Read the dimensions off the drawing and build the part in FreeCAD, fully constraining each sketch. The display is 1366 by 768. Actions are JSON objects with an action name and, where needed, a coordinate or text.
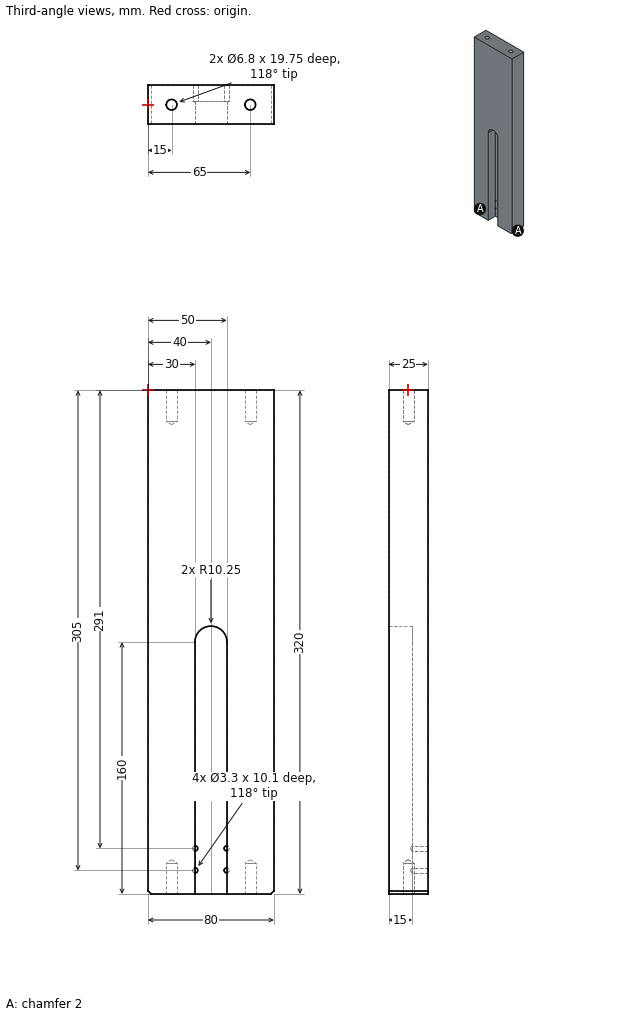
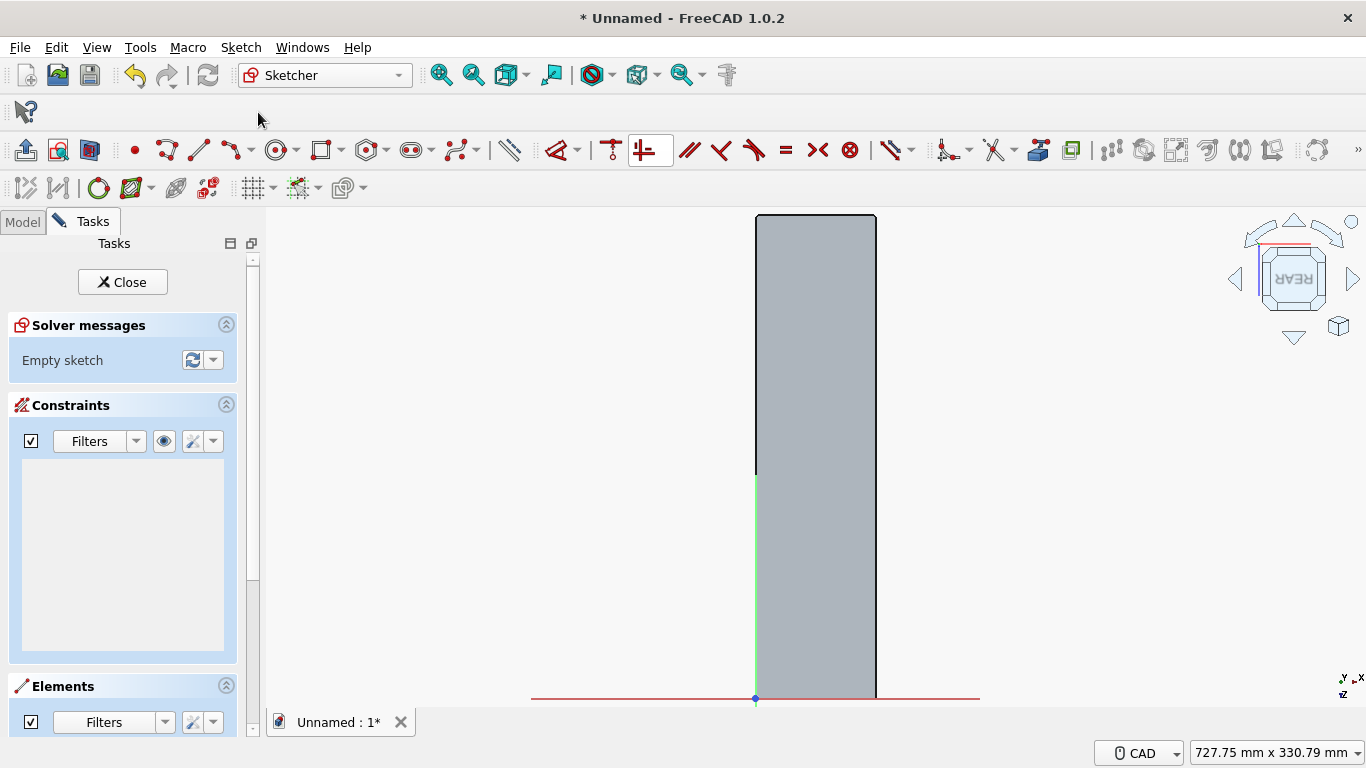
{"action": "scroll", "coordinate": [748, 457], "scroll_direction": "down", "scroll_amount": 5}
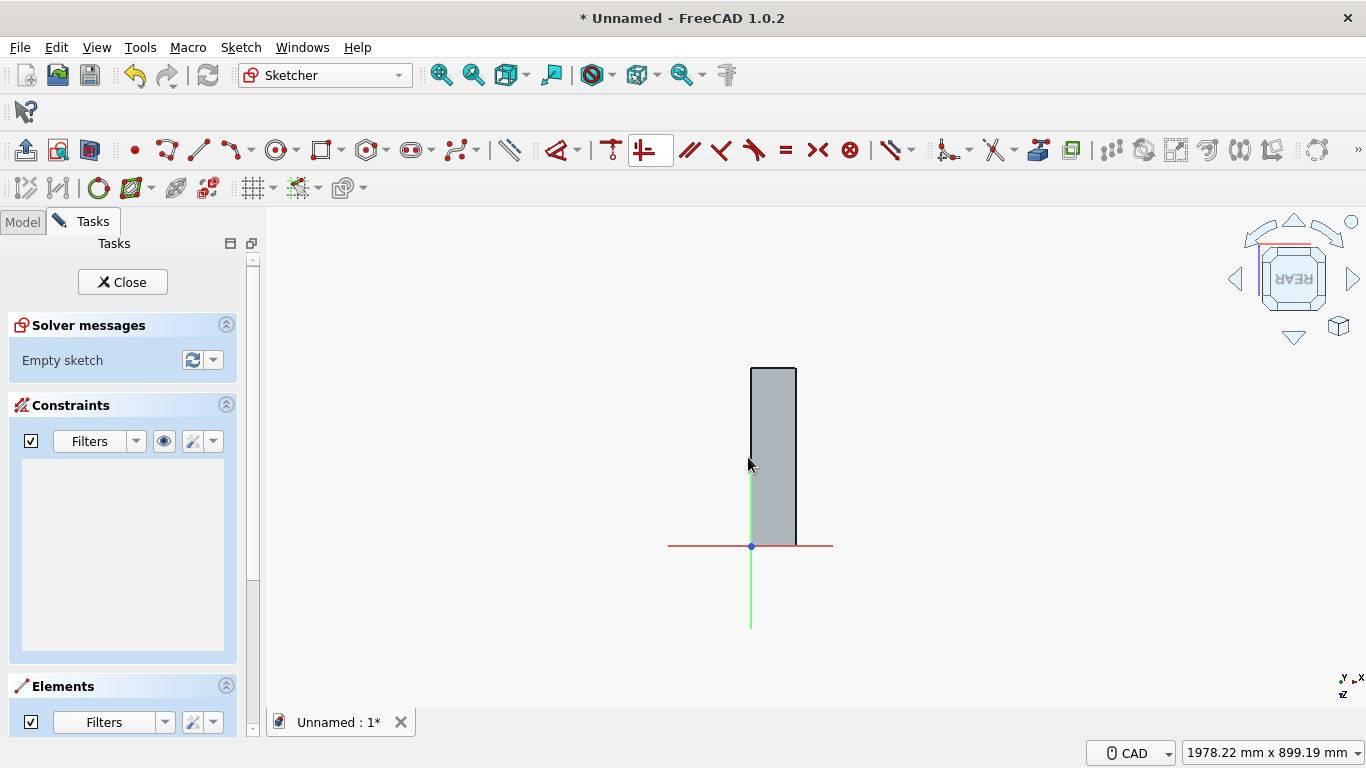
{"action": "scroll", "coordinate": [775, 377], "scroll_direction": "up", "scroll_amount": 15}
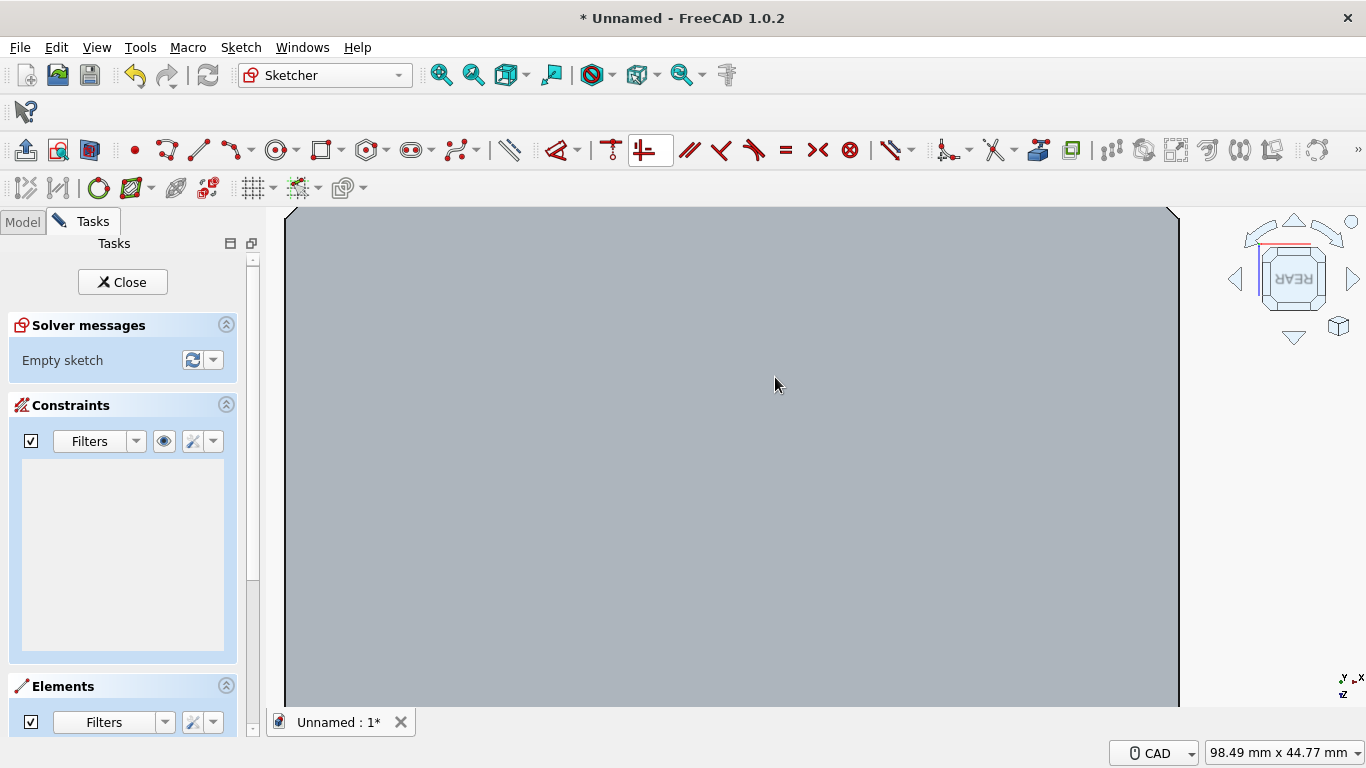
{"action": "scroll", "coordinate": [700, 413], "scroll_direction": "up", "scroll_amount": 2}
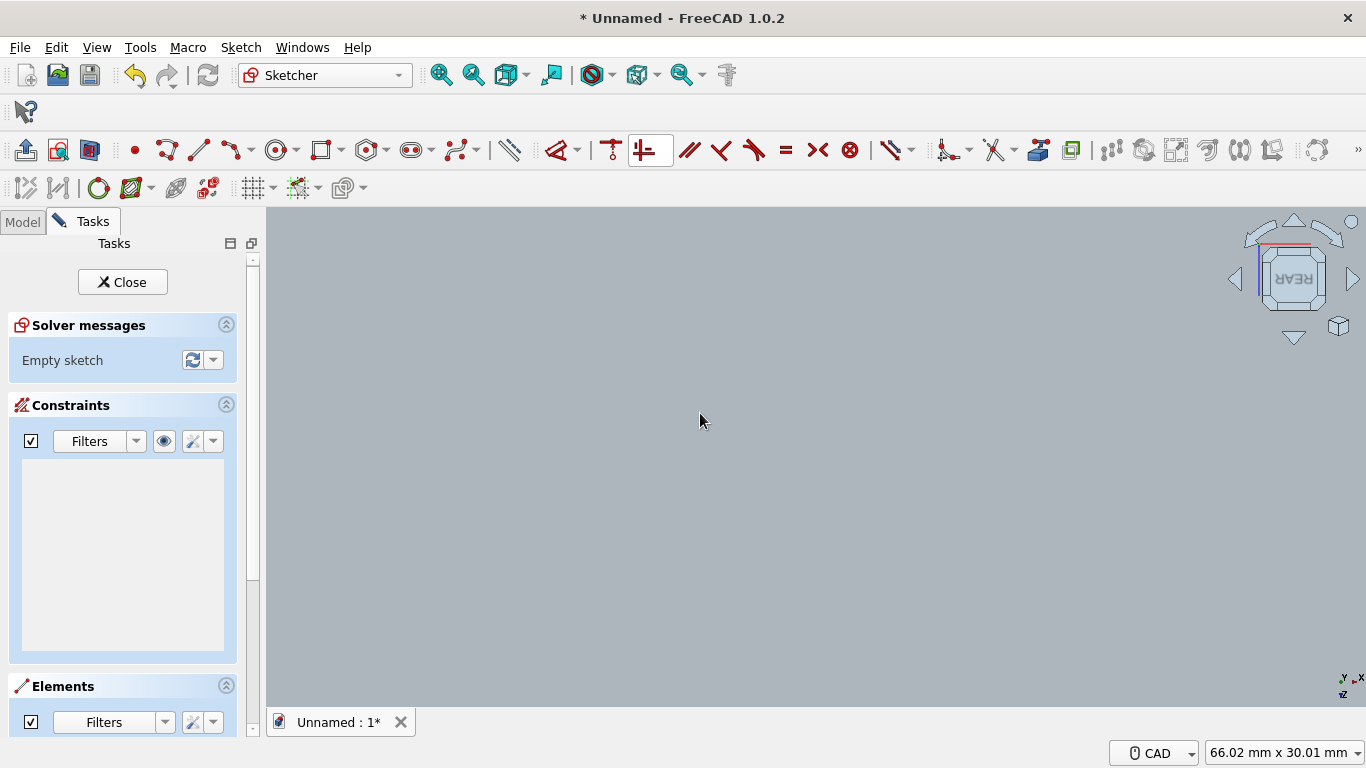
{"action": "left_click", "coordinate": [276, 150]}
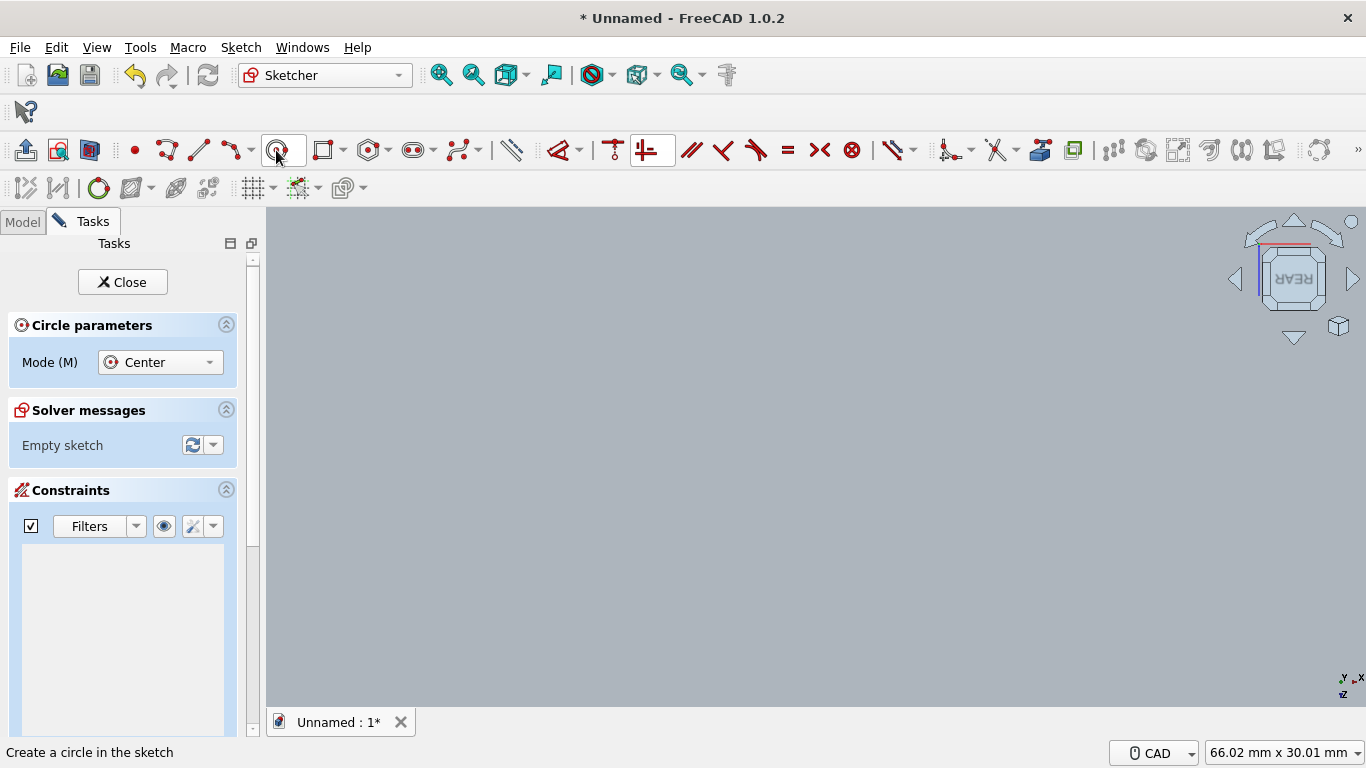
{"action": "left_click", "coordinate": [581, 340]}
{"action": "mouse_move", "coordinate": [600, 321]}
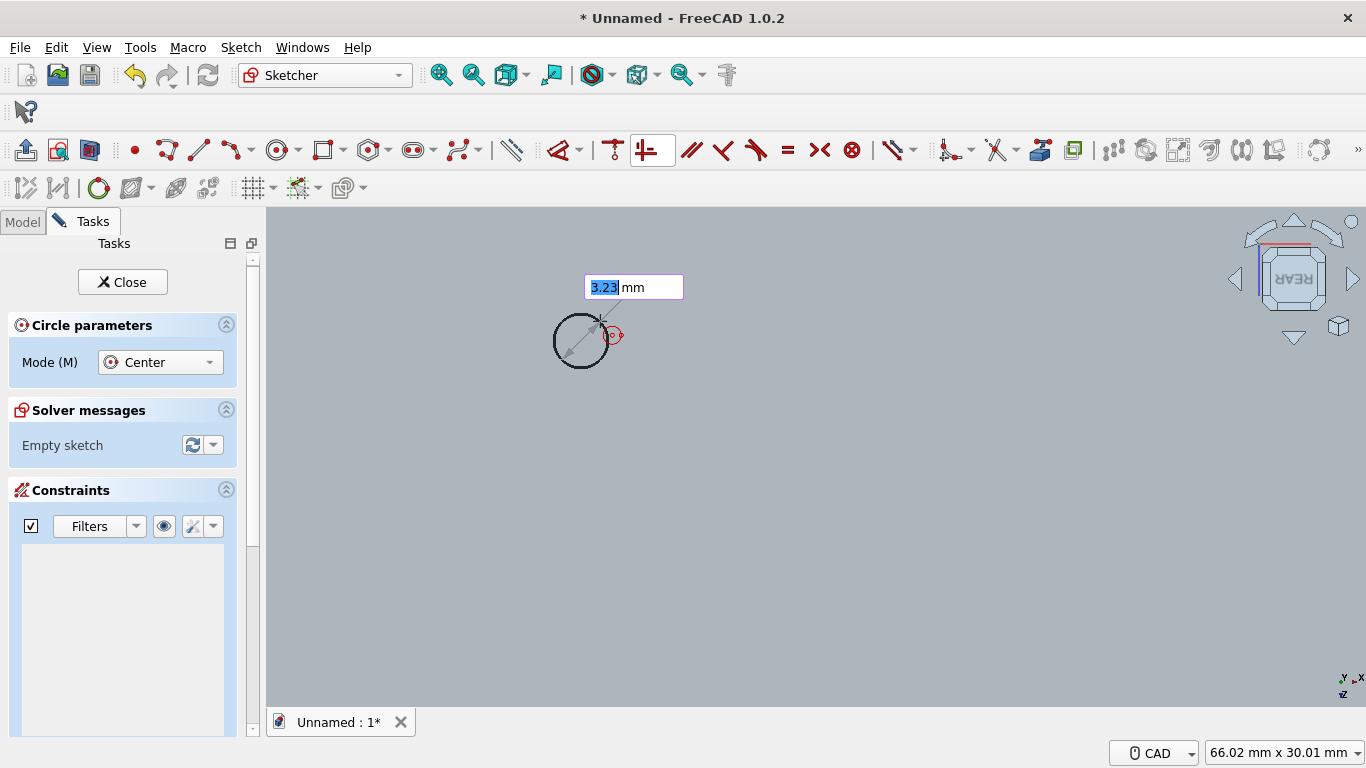
{"action": "type", "text": "3.3"}
{"action": "key", "text": "Return"}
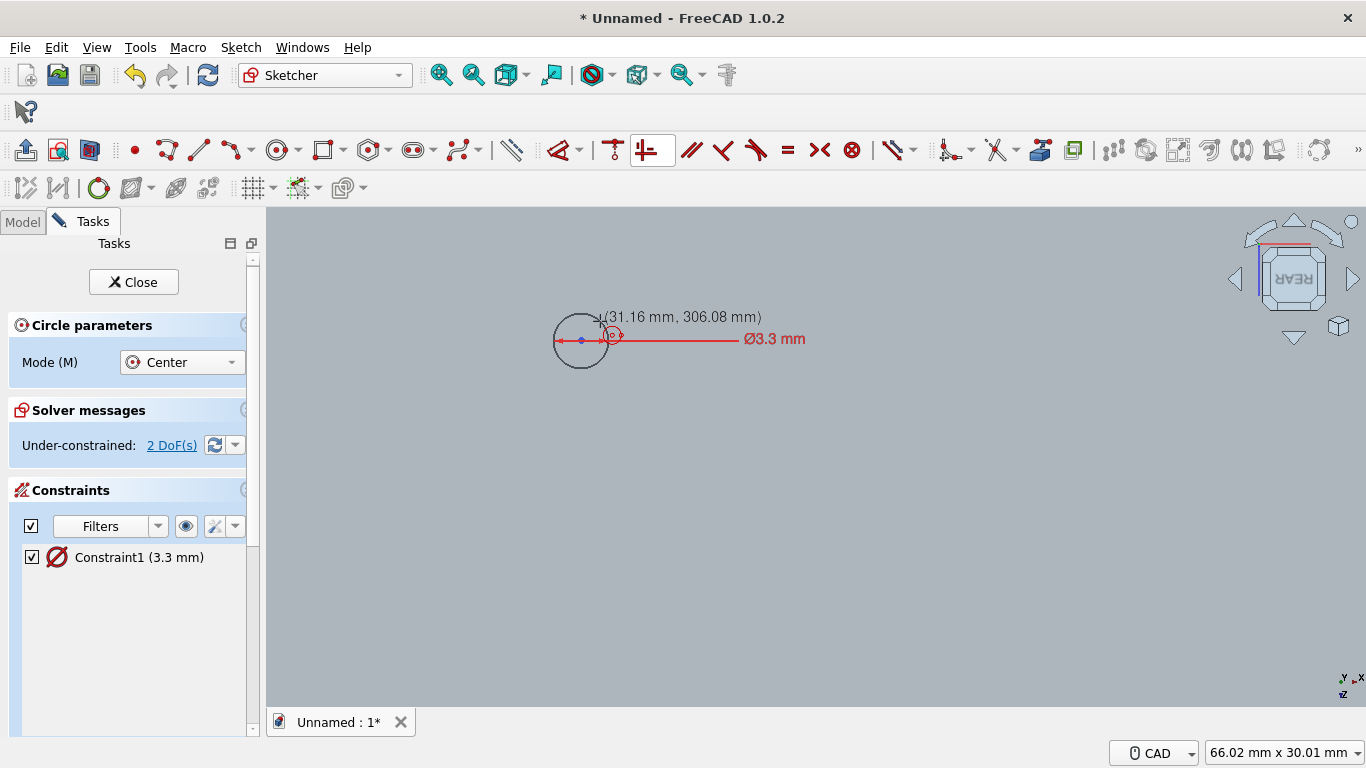
{"action": "left_click", "coordinate": [581, 573]}
{"action": "mouse_move", "coordinate": [600, 554]}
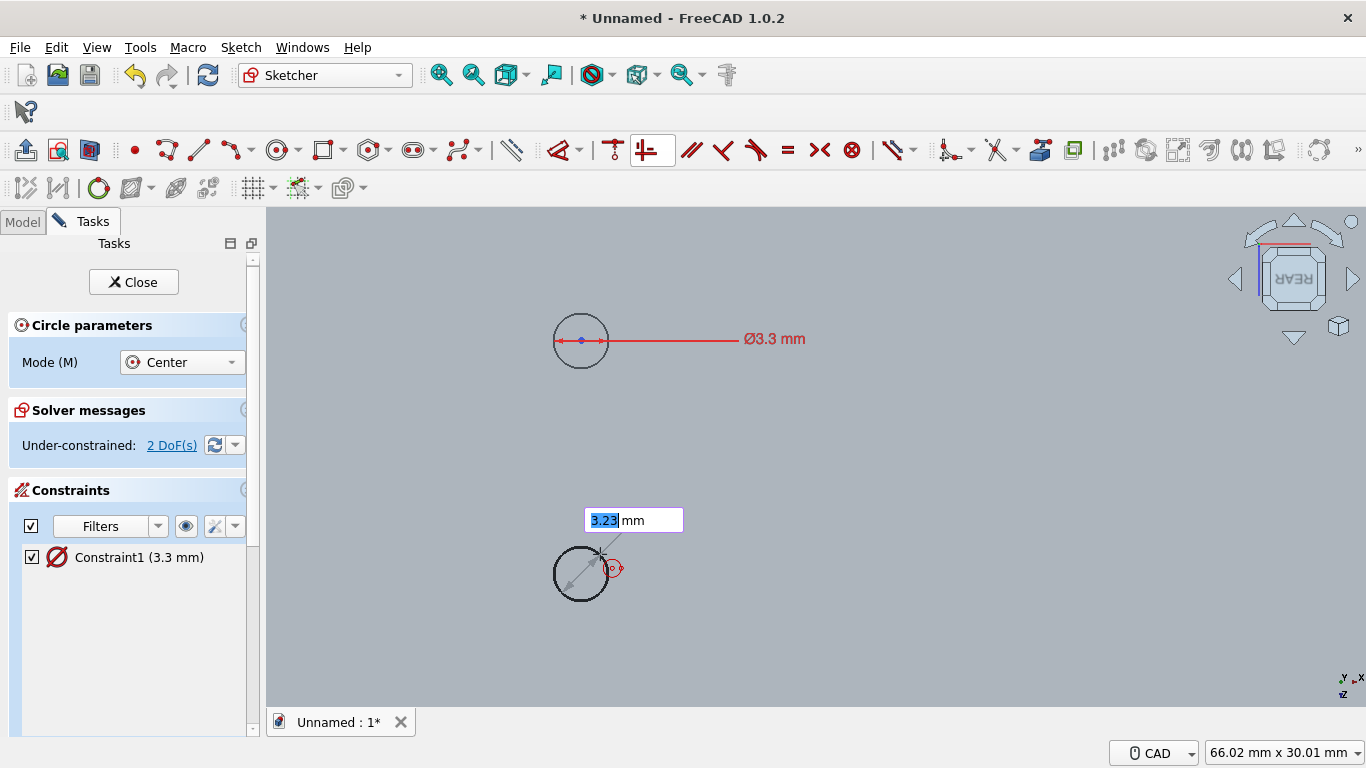
{"action": "type", "text": "3.3"}
{"action": "key", "text": "Return"}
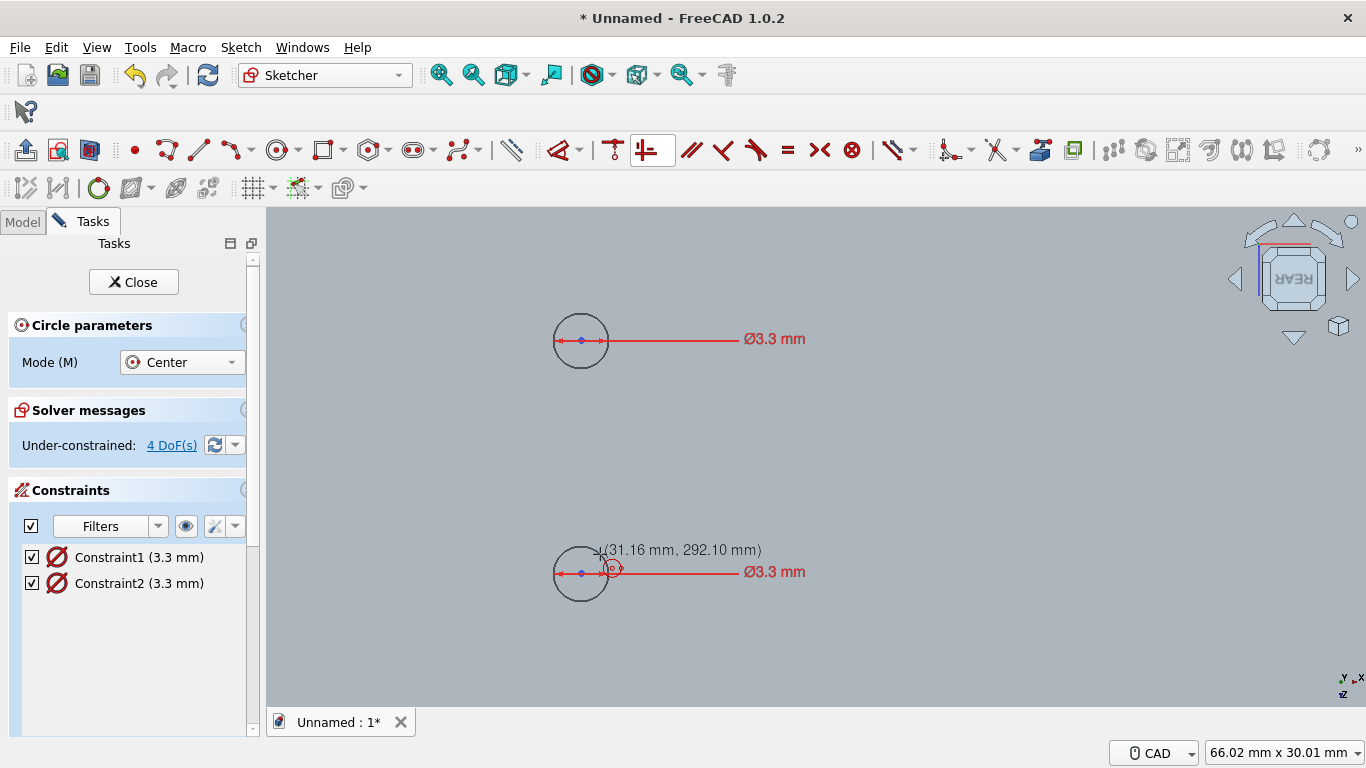
{"action": "left_click", "coordinate": [914, 573]}
{"action": "mouse_move", "coordinate": [933, 554]}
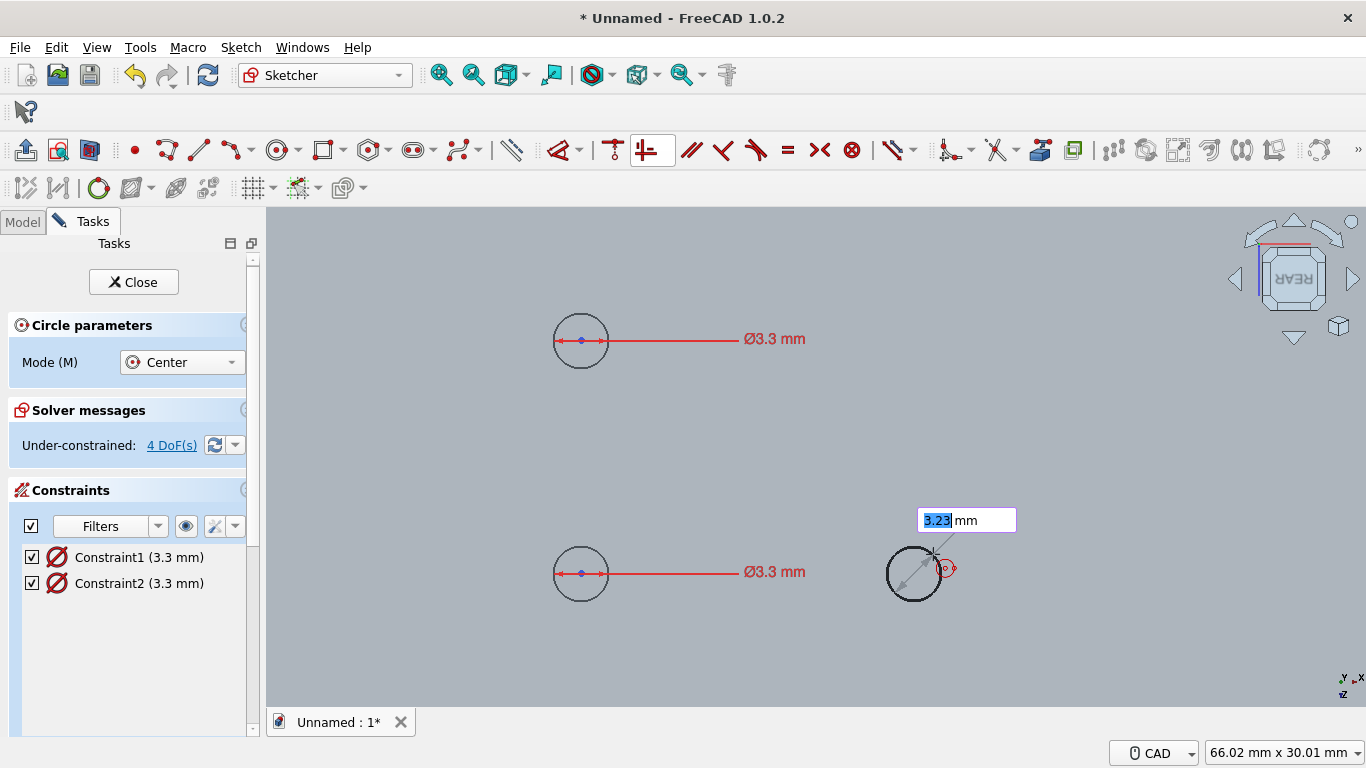
{"action": "type", "text": "3.3"}
{"action": "key", "text": "Return"}